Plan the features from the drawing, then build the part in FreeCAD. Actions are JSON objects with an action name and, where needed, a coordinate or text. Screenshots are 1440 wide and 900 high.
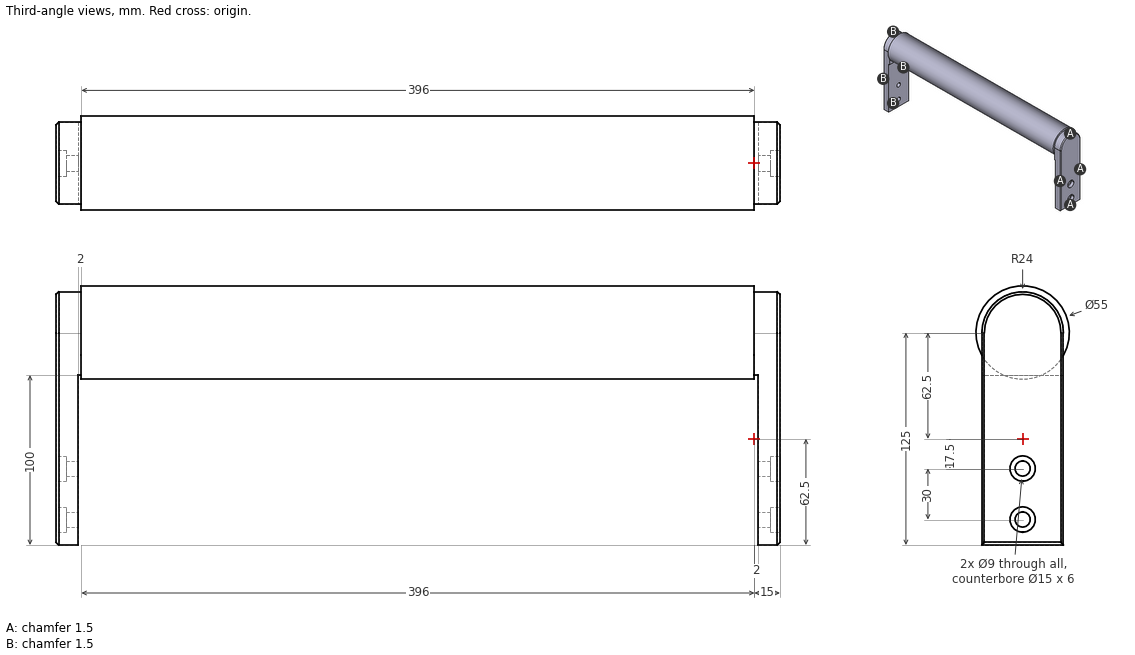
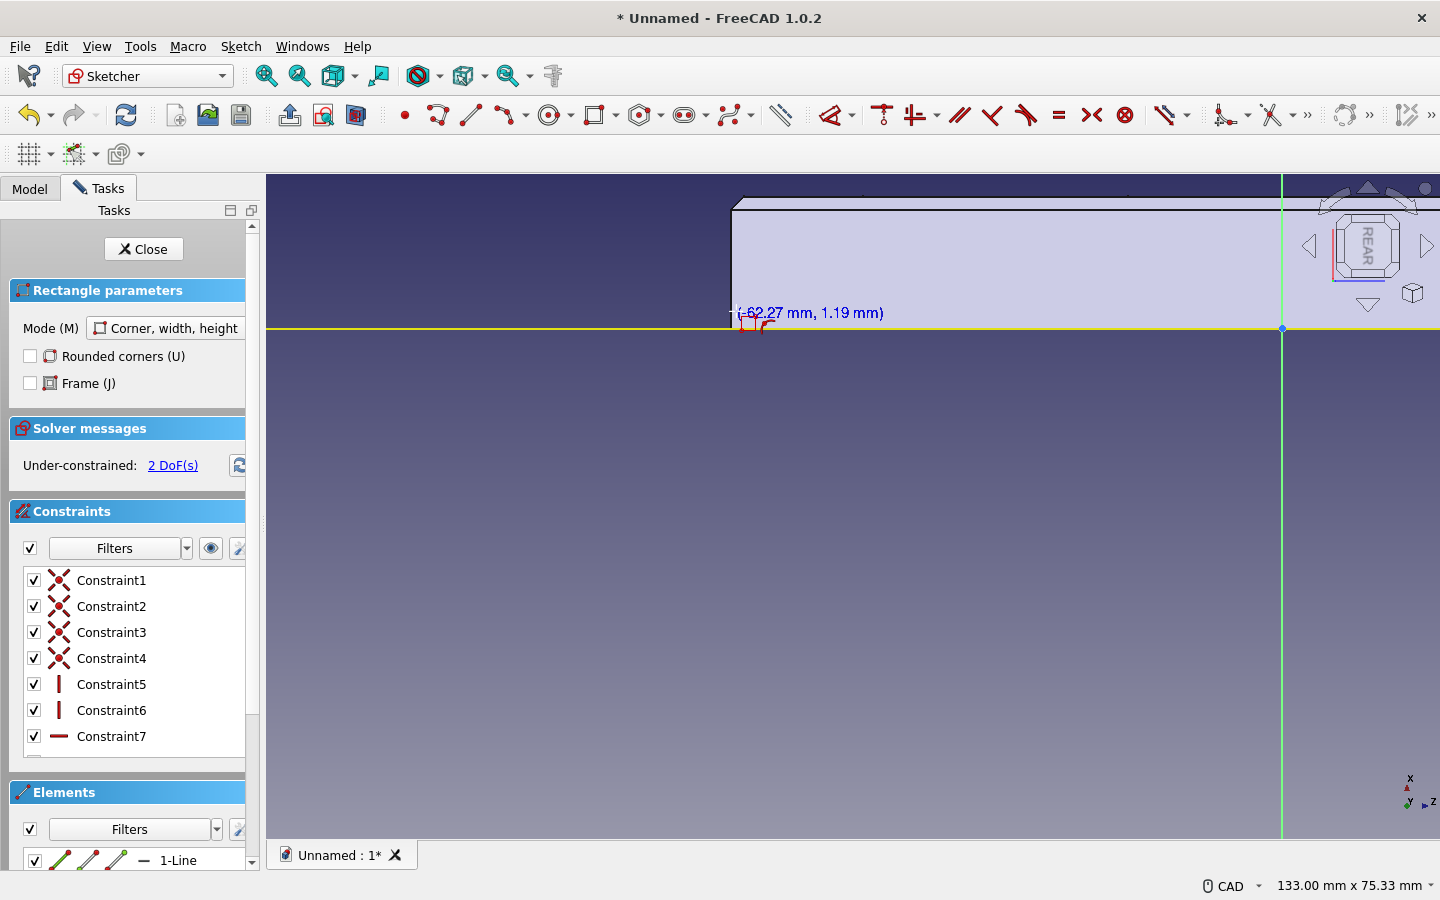
{"action": "left_click", "coordinate": [731, 311]}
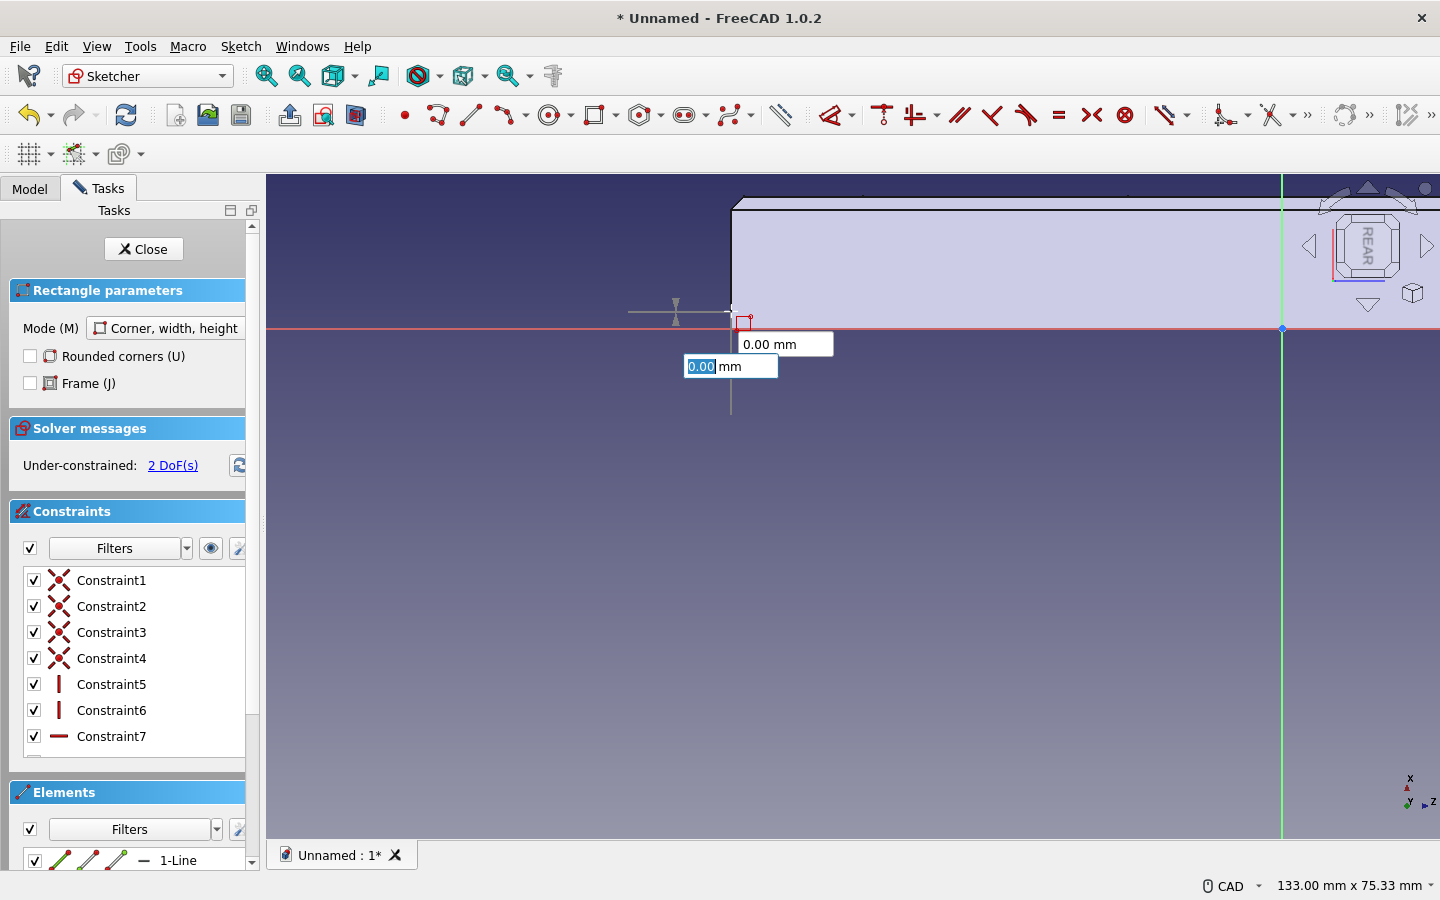
{"action": "scroll", "coordinate": [736, 311], "scroll_direction": "down", "scroll_amount": 11}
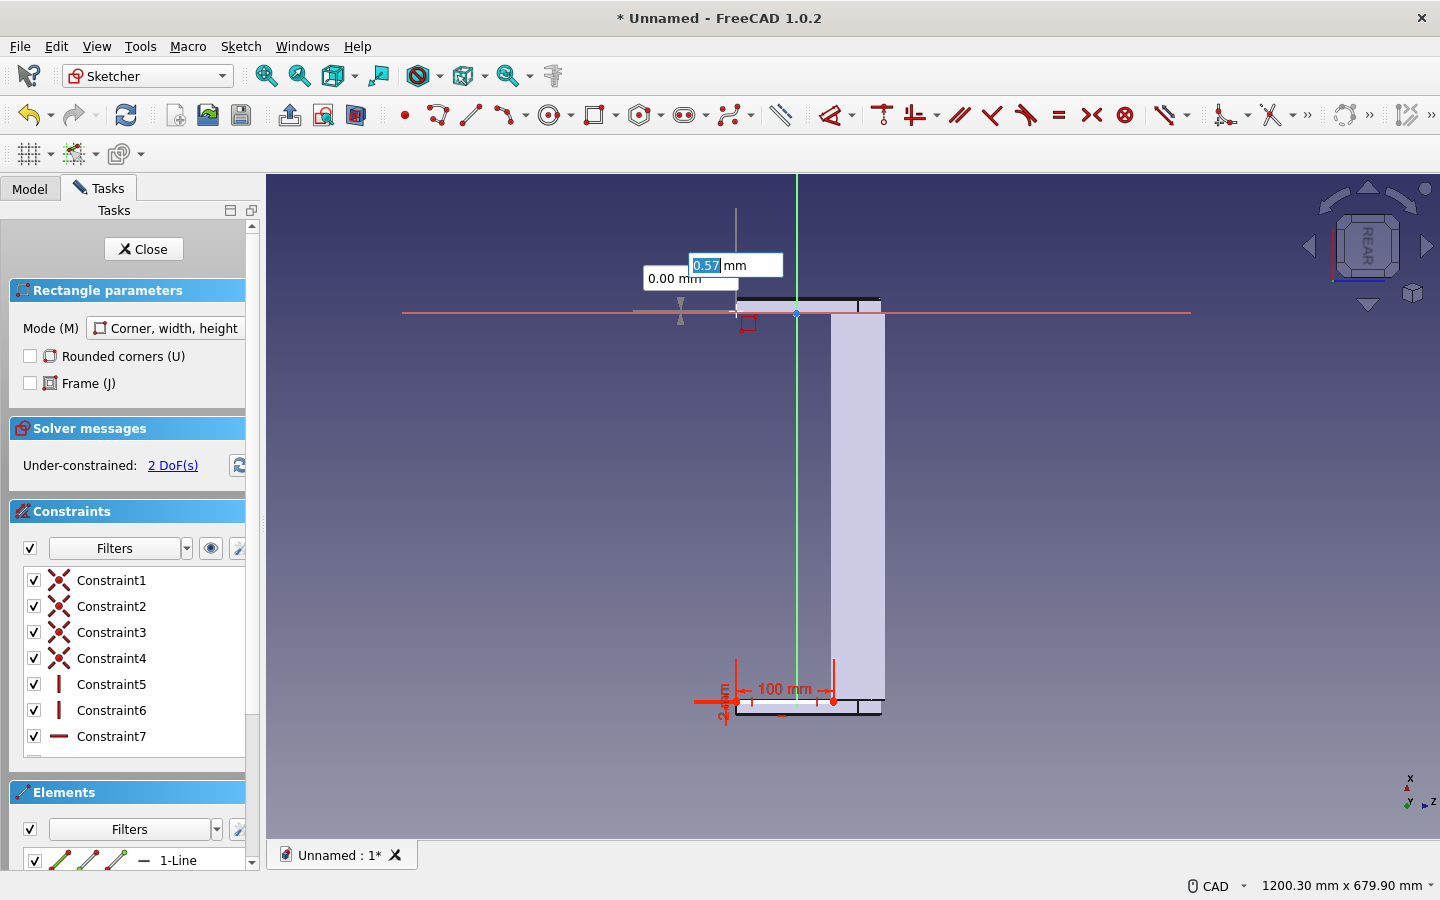
{"action": "left_click", "coordinate": [834, 313]}
{"action": "key", "text": "Escape"}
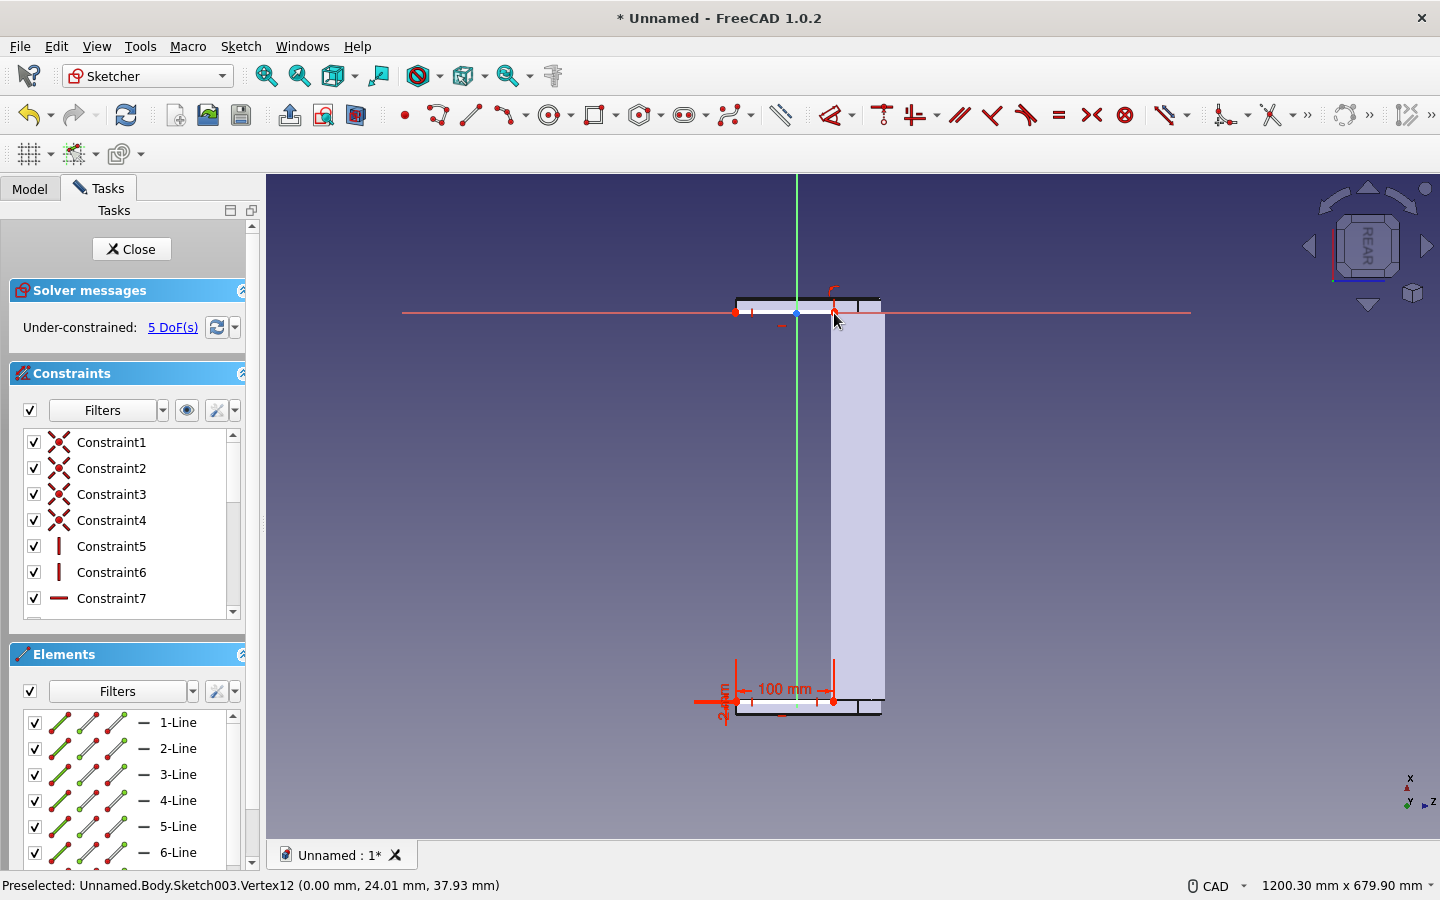
{"action": "left_click", "coordinate": [830, 116]}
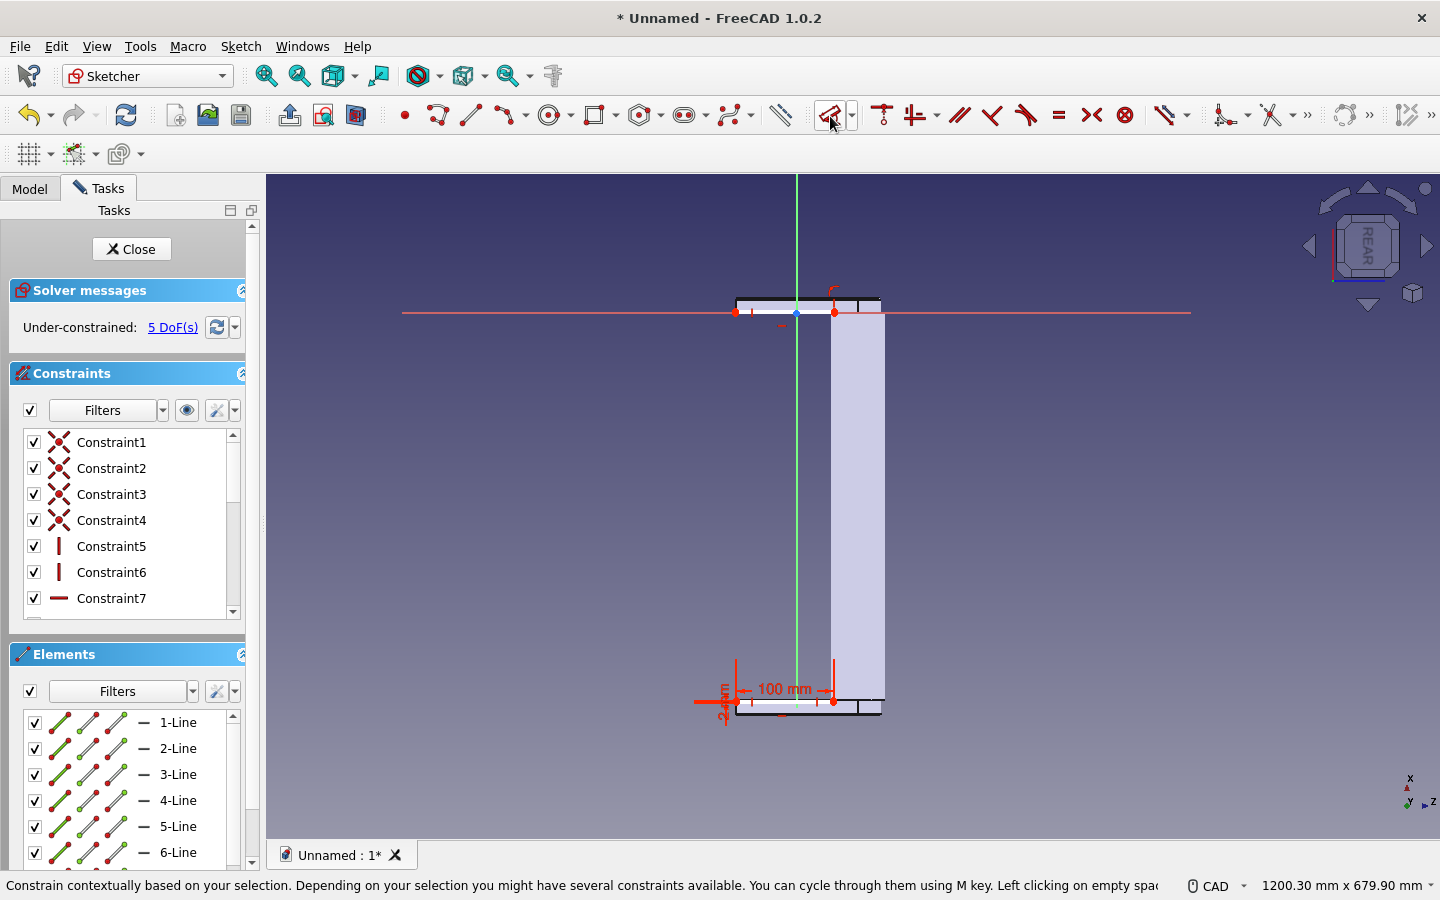
{"action": "scroll", "coordinate": [736, 312], "scroll_direction": "up", "scroll_amount": 16}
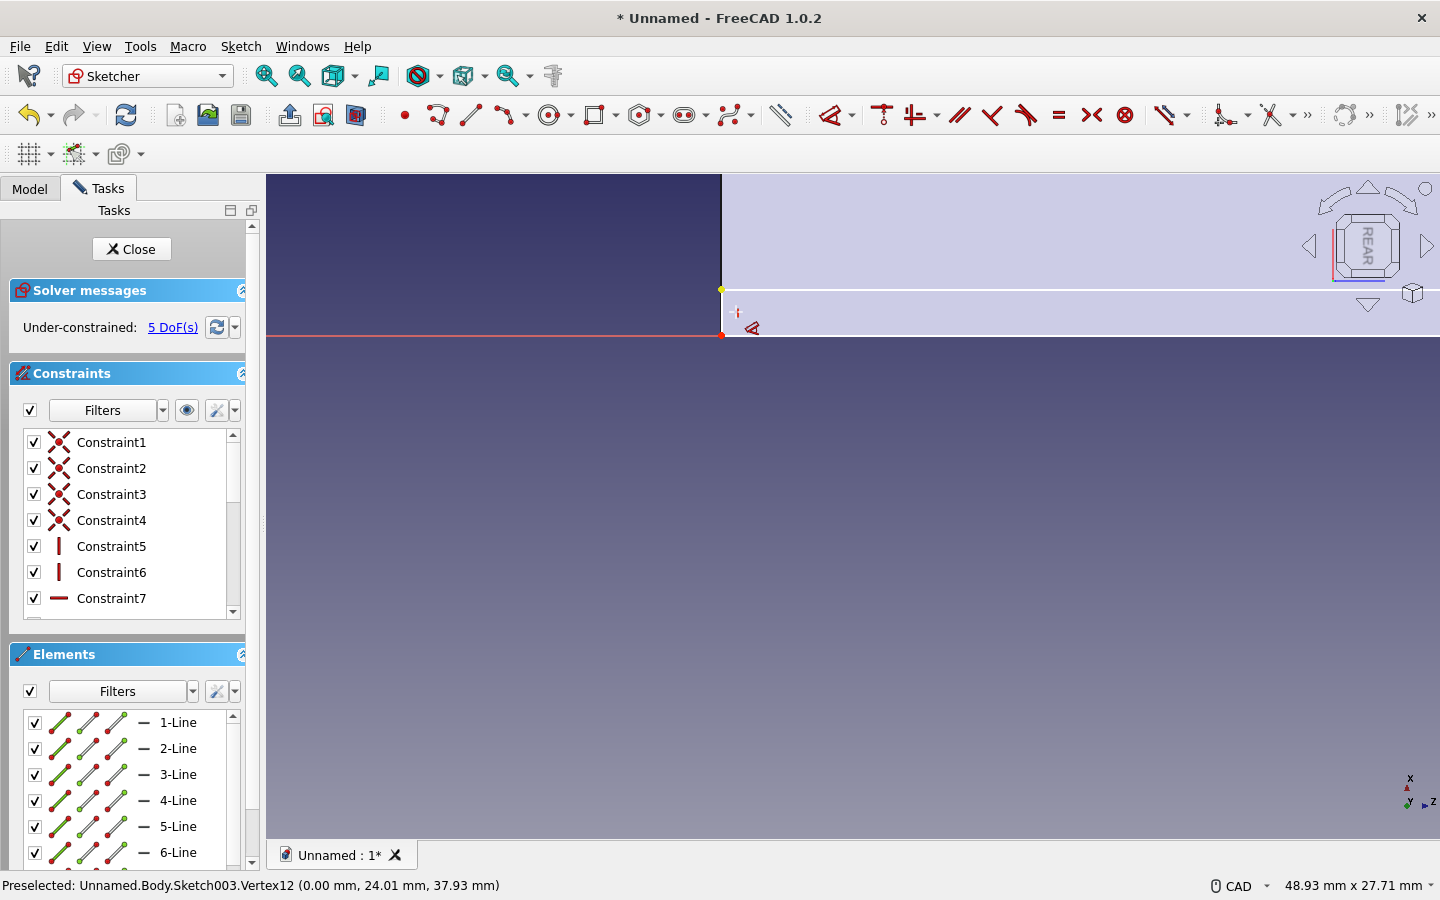
{"action": "left_click", "coordinate": [722, 313]}
{"action": "left_click", "coordinate": [688, 313]}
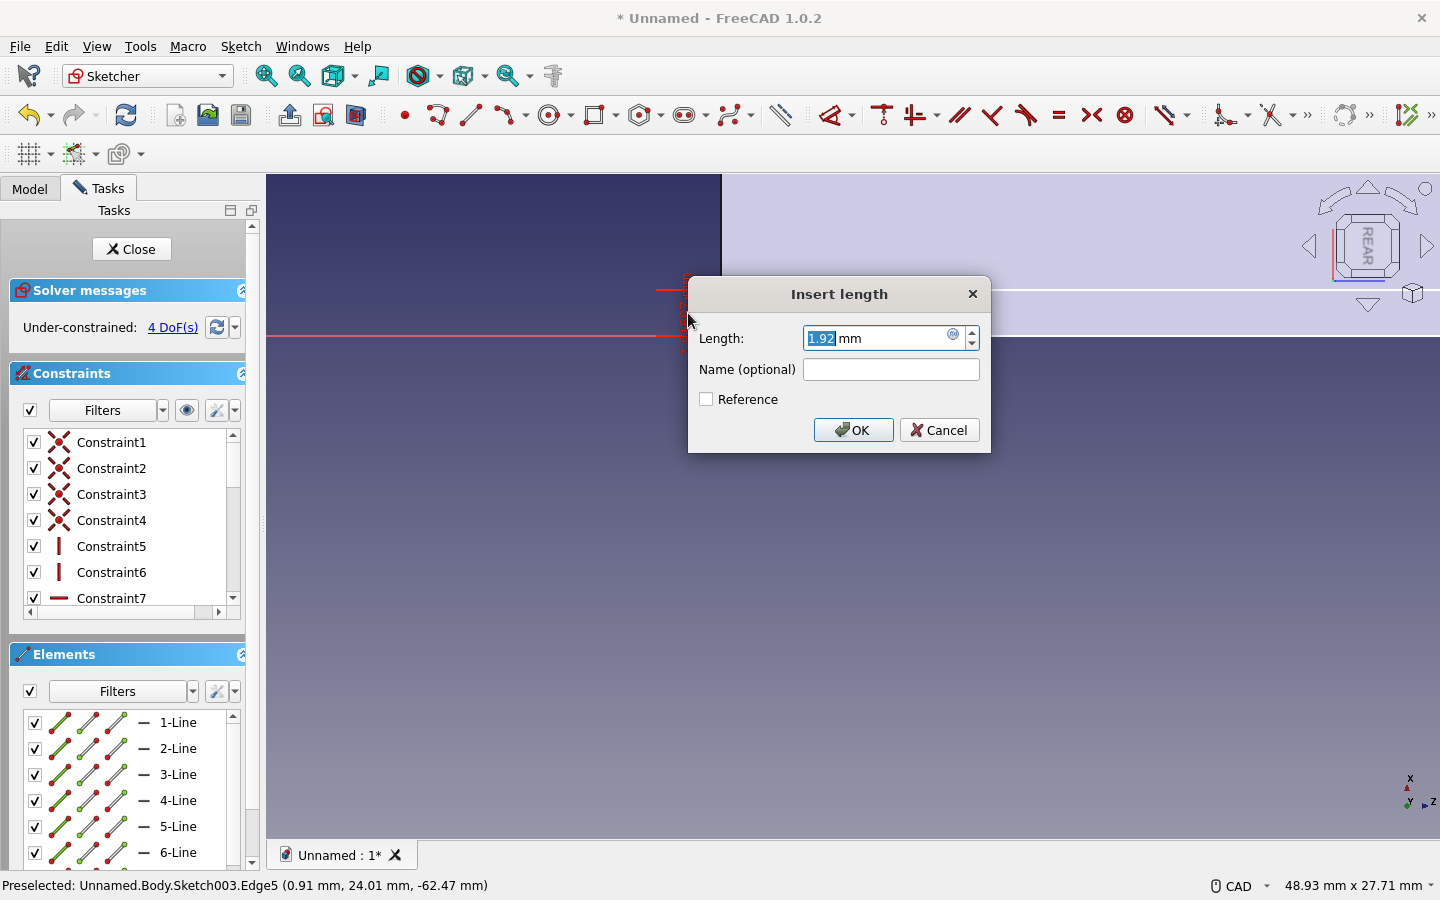
{"action": "type", "text": "2"}
{"action": "key", "text": "Return"}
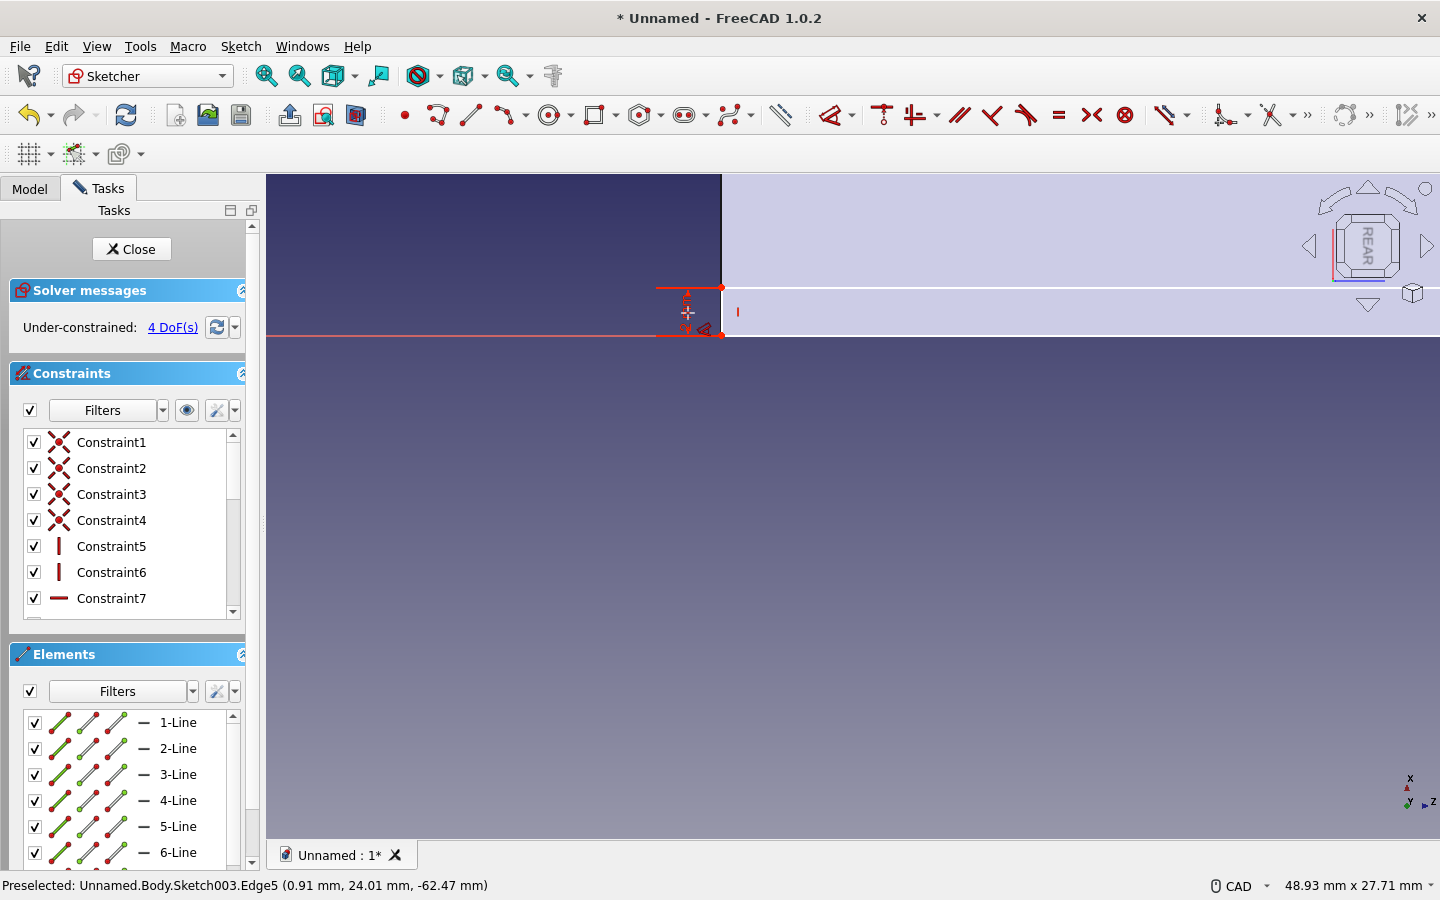
{"action": "scroll", "coordinate": [725, 267], "scroll_direction": "down", "scroll_amount": 15}